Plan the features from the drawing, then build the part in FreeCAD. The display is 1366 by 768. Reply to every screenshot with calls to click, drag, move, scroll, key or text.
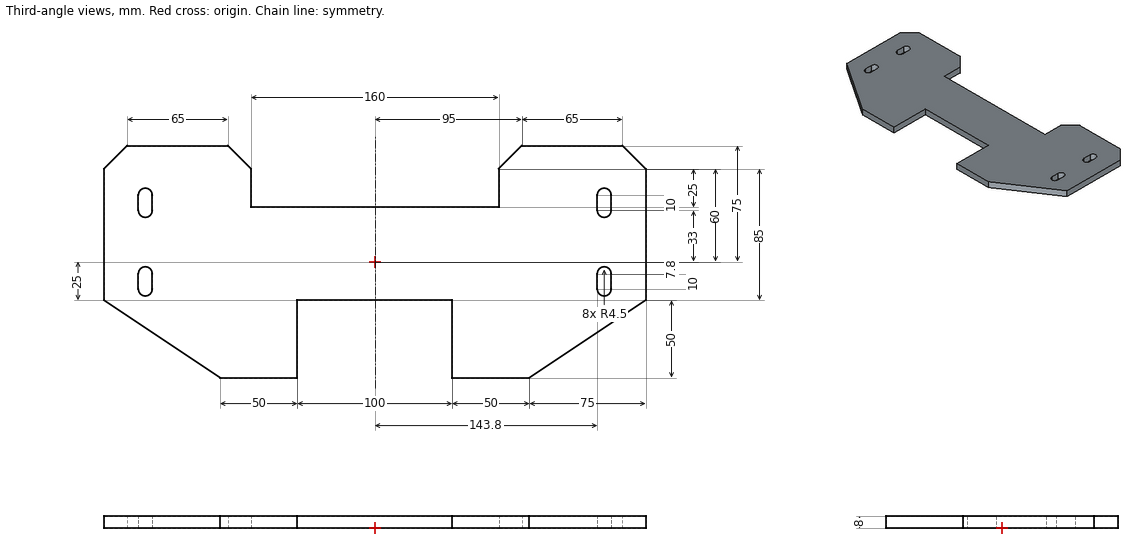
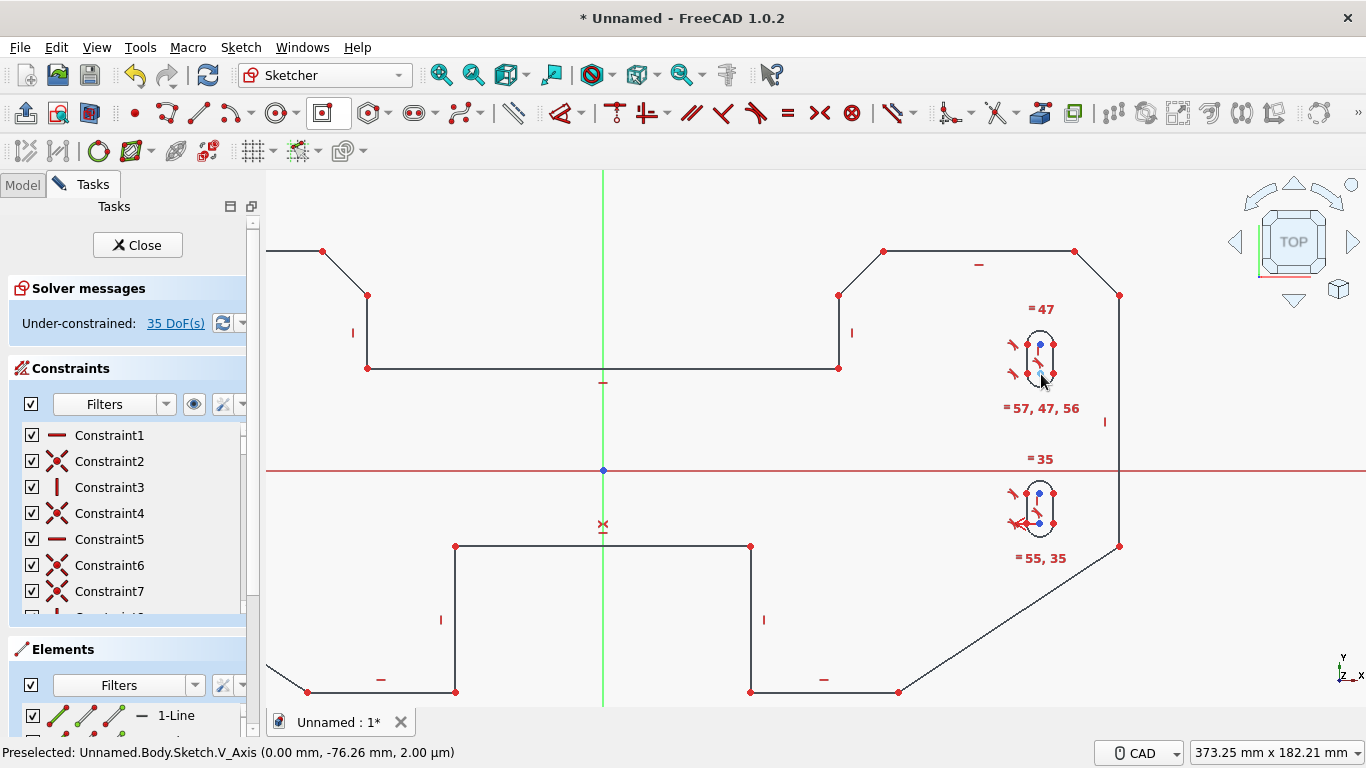
click(1040, 374)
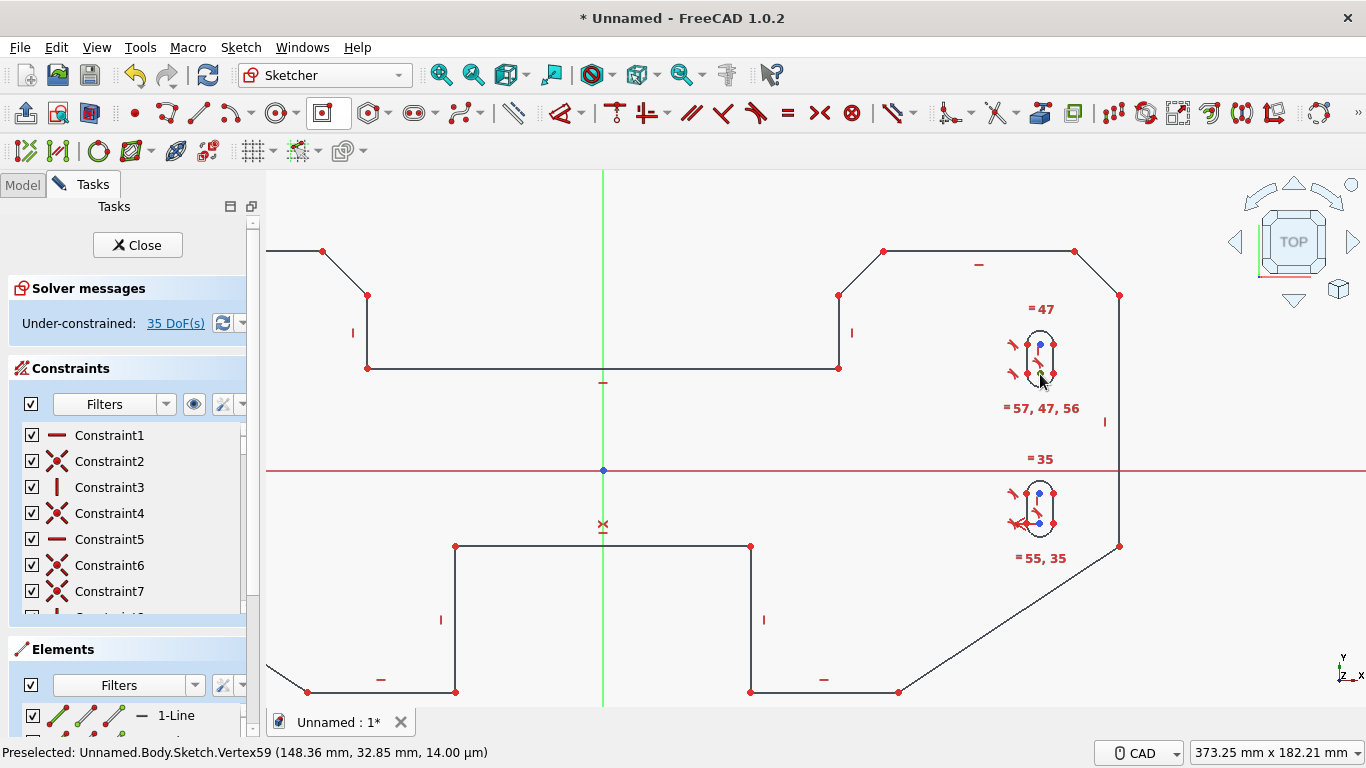
scroll(1041, 373, down, 2)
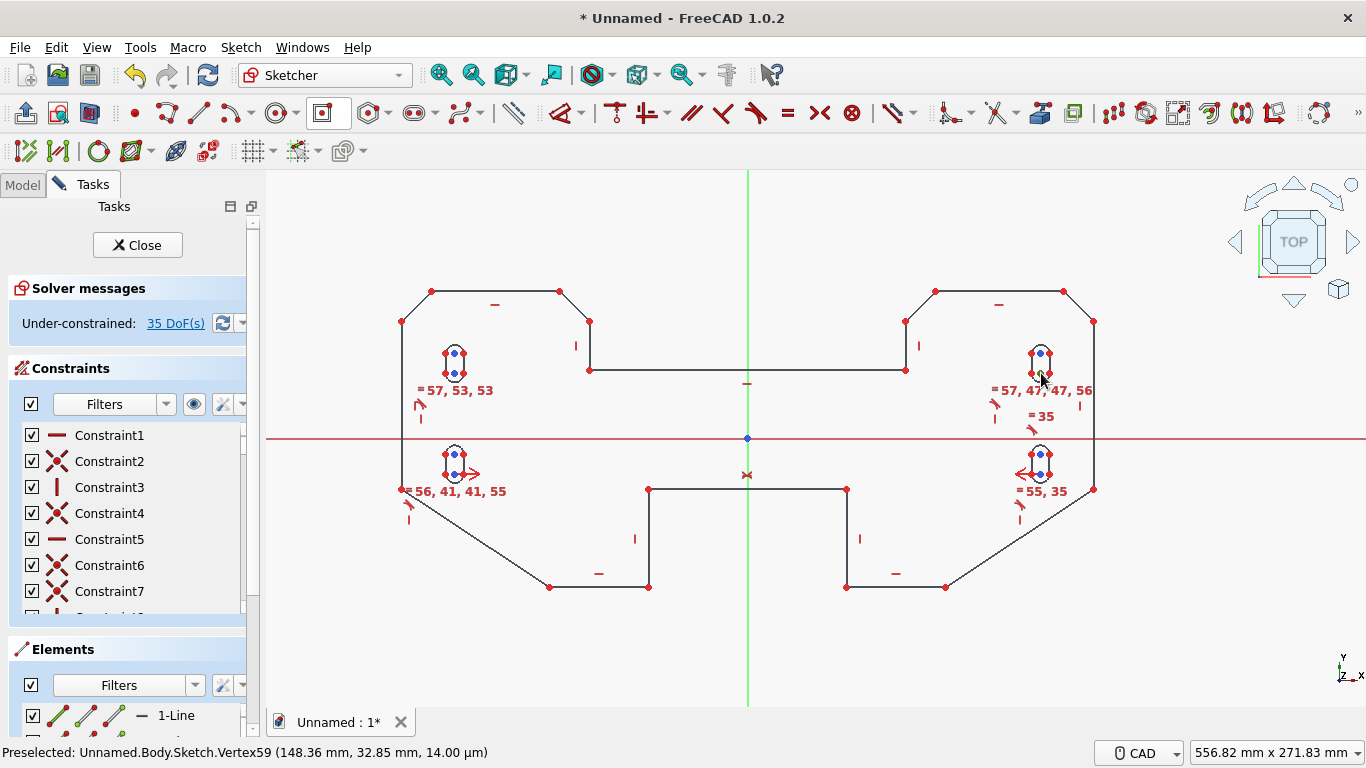
scroll(455, 374, up, 2)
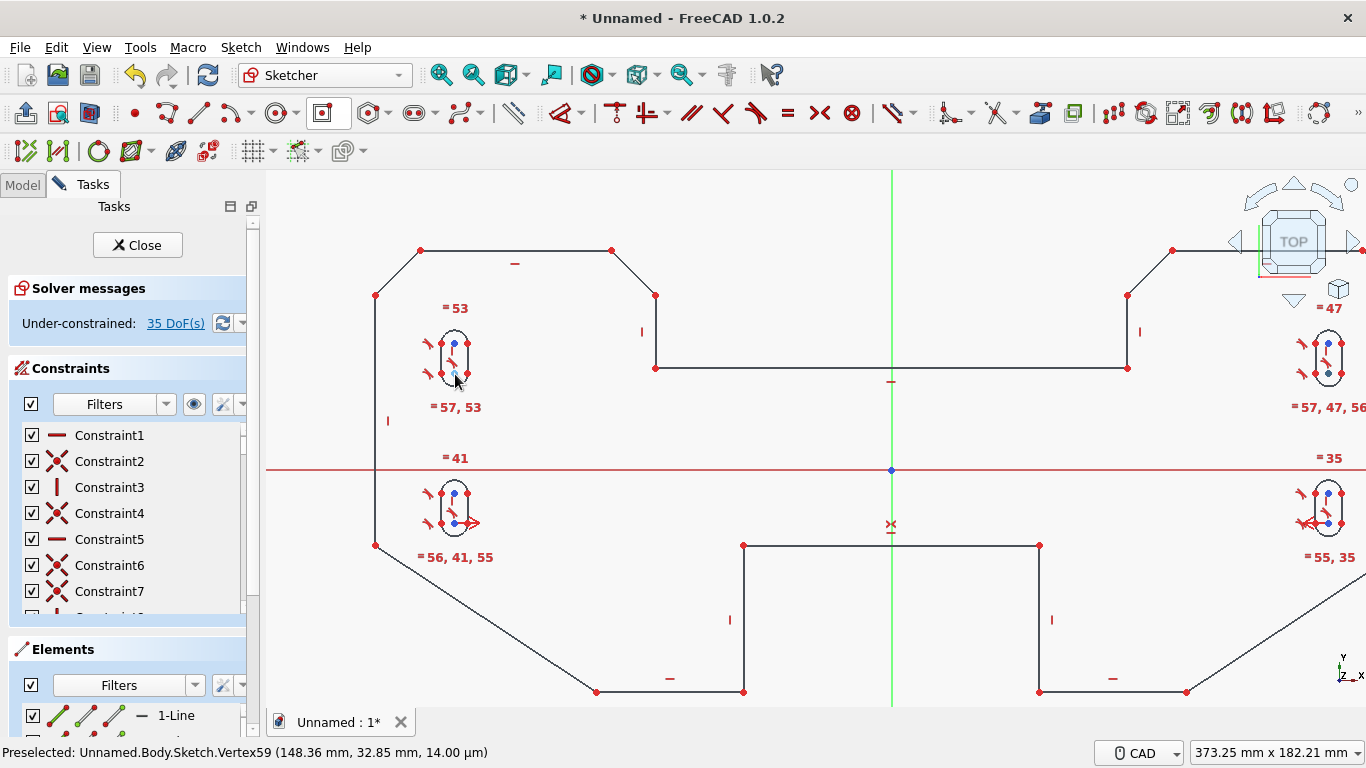
click(455, 373)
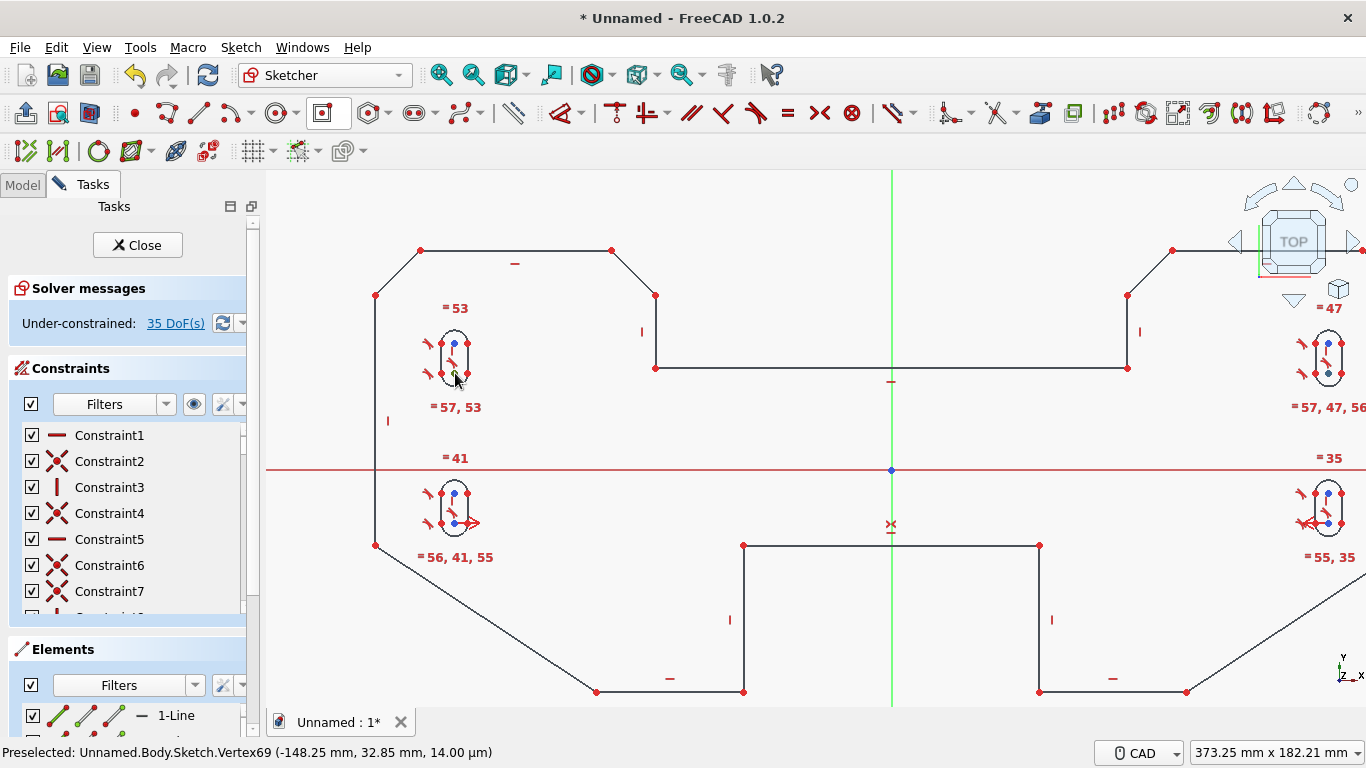
click(892, 645)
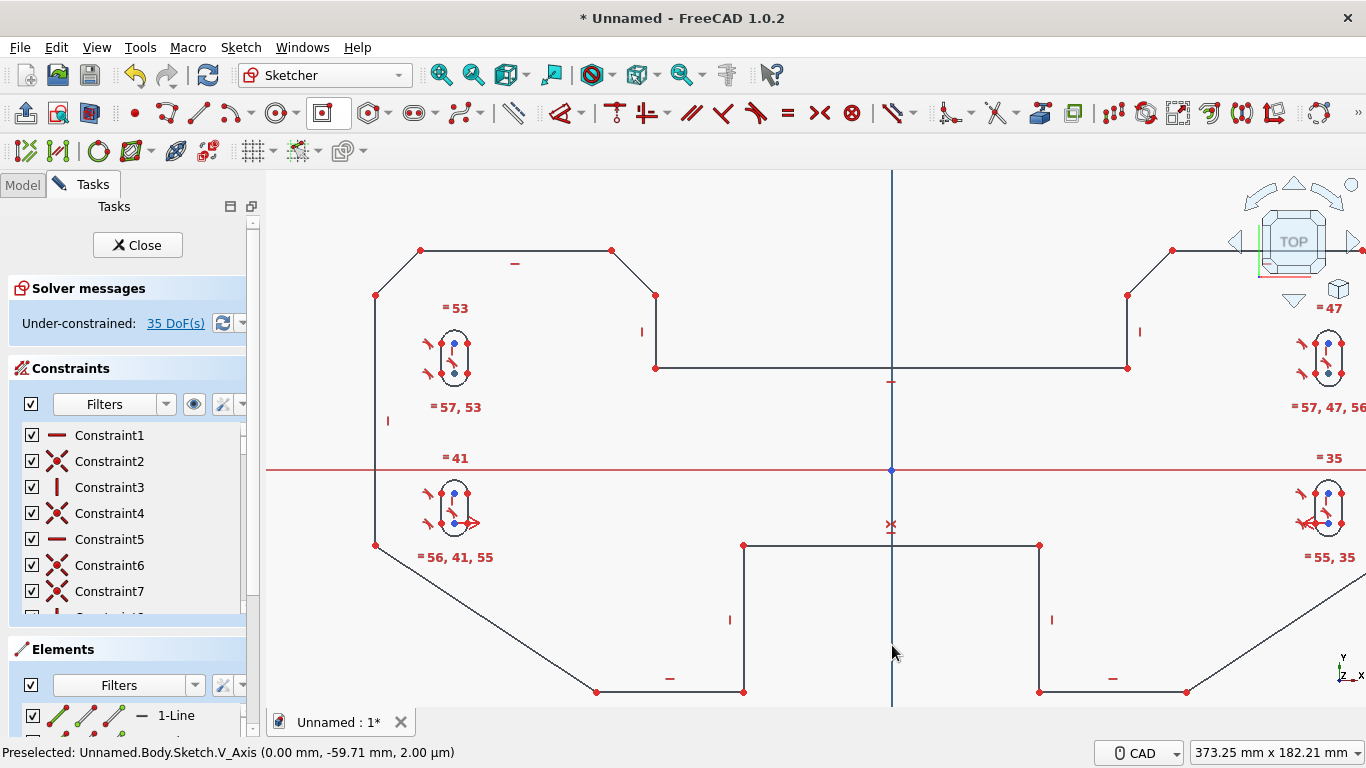
click(820, 114)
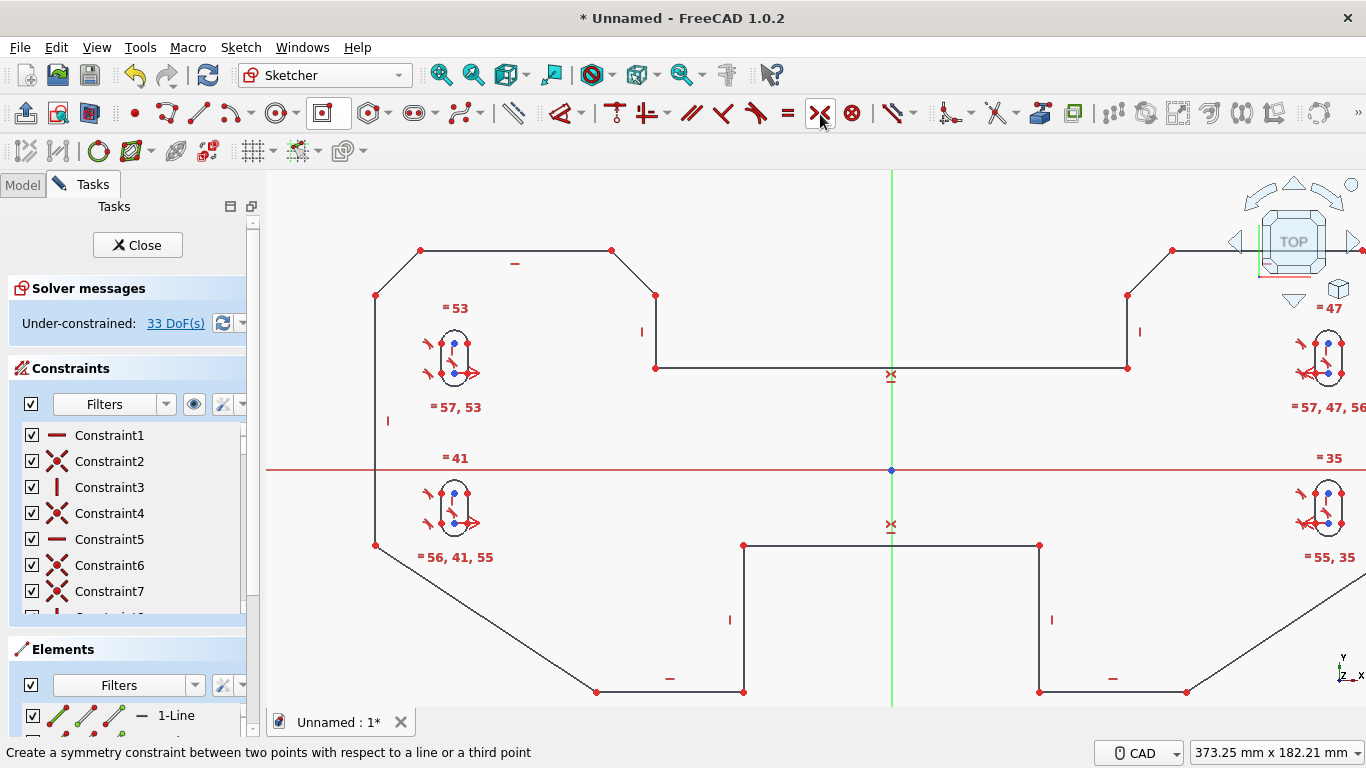
click(1127, 295)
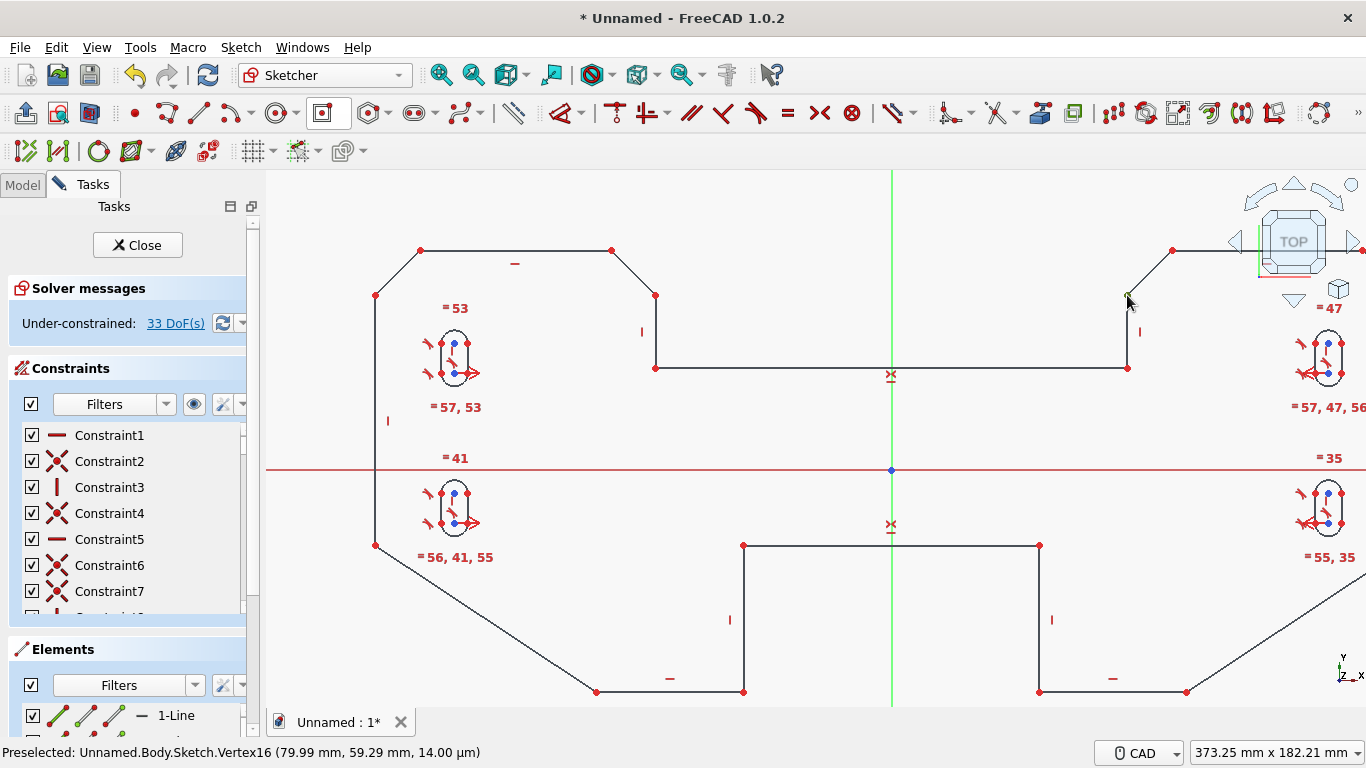
click(656, 295)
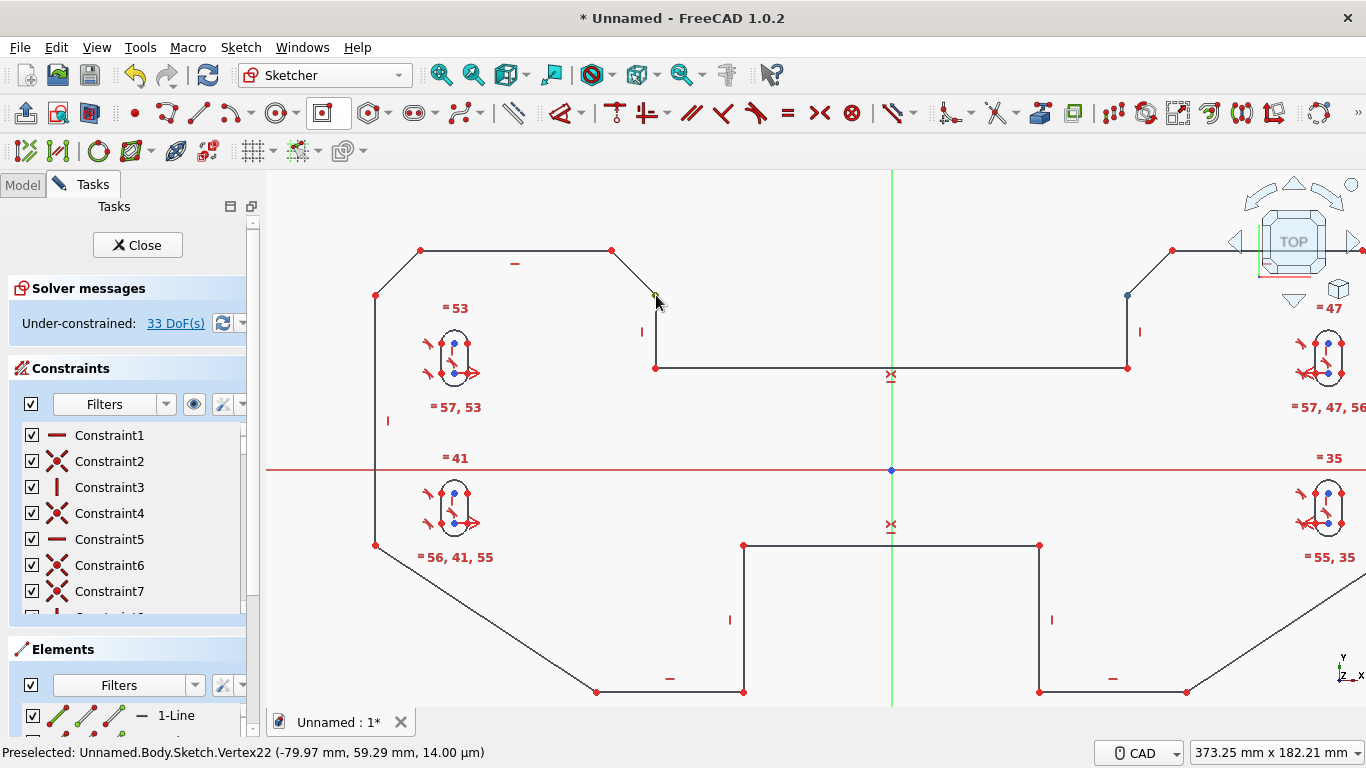
click(892, 645)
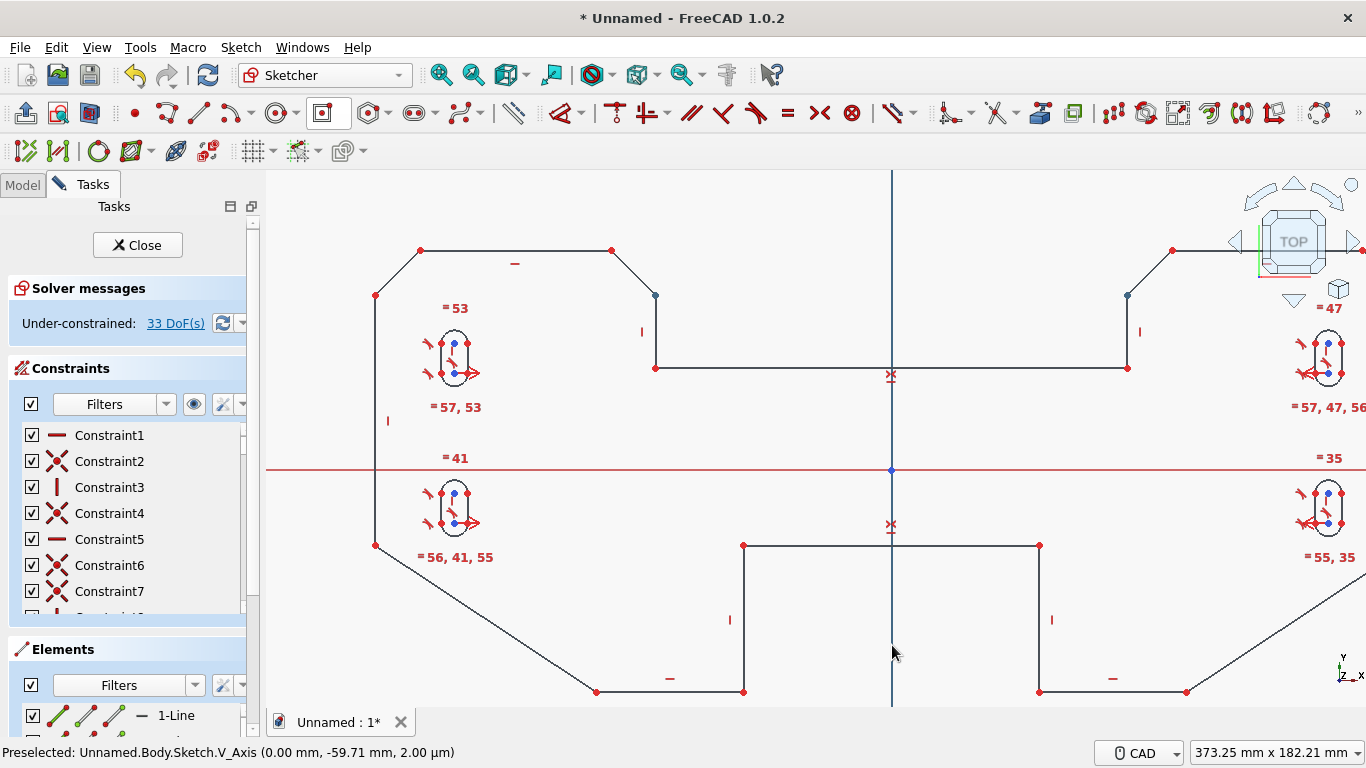
click(820, 114)